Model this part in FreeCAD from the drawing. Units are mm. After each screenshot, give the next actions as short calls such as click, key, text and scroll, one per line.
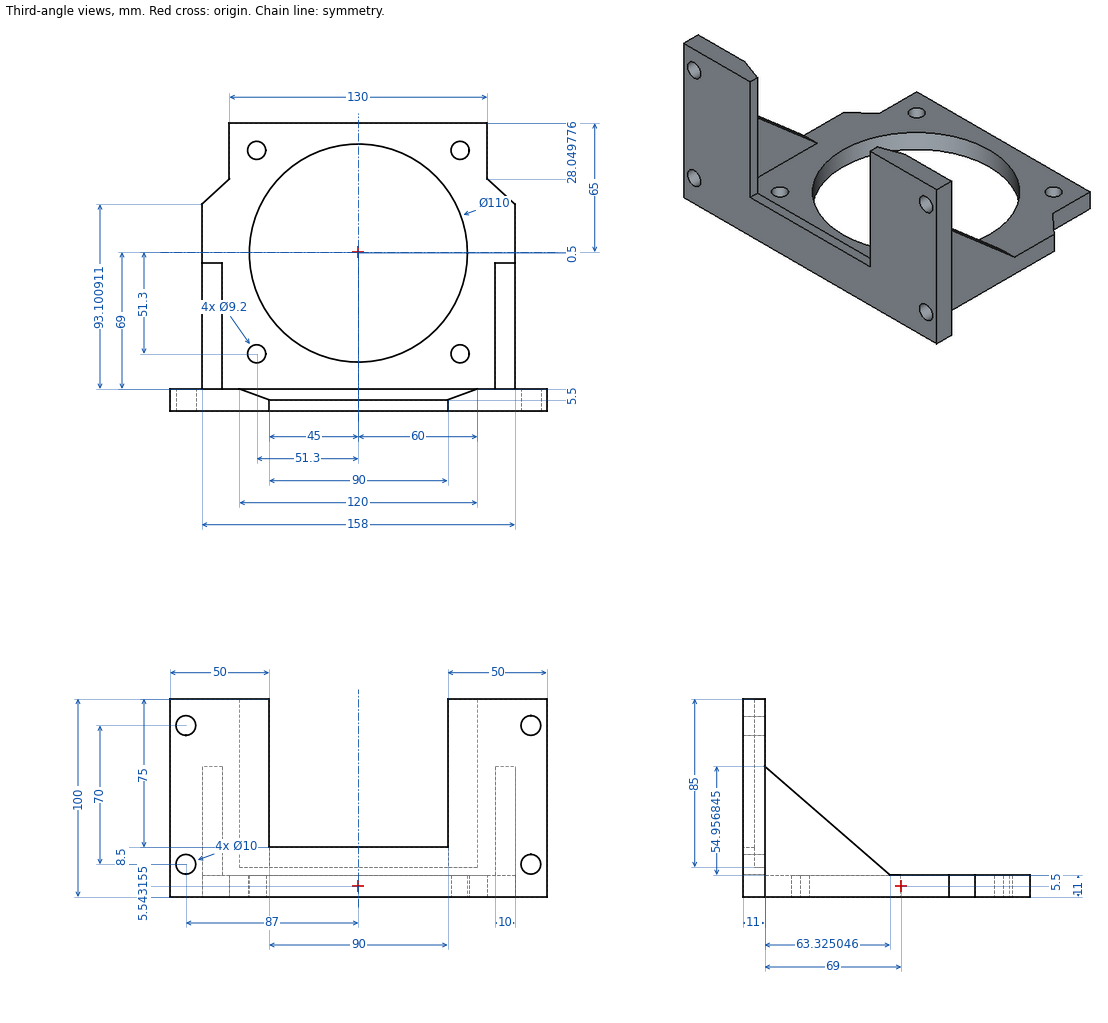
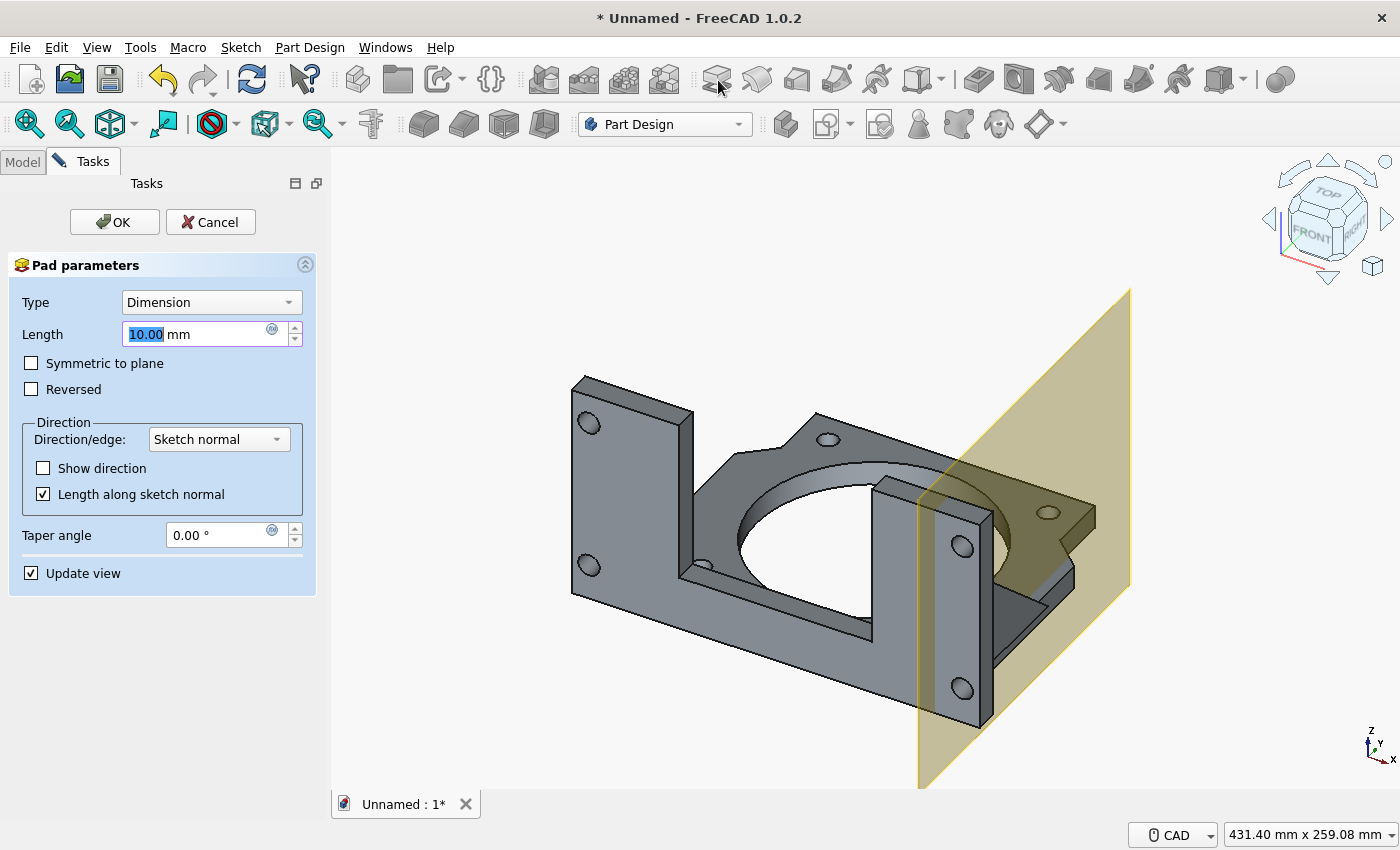
text(10)
key(Tab)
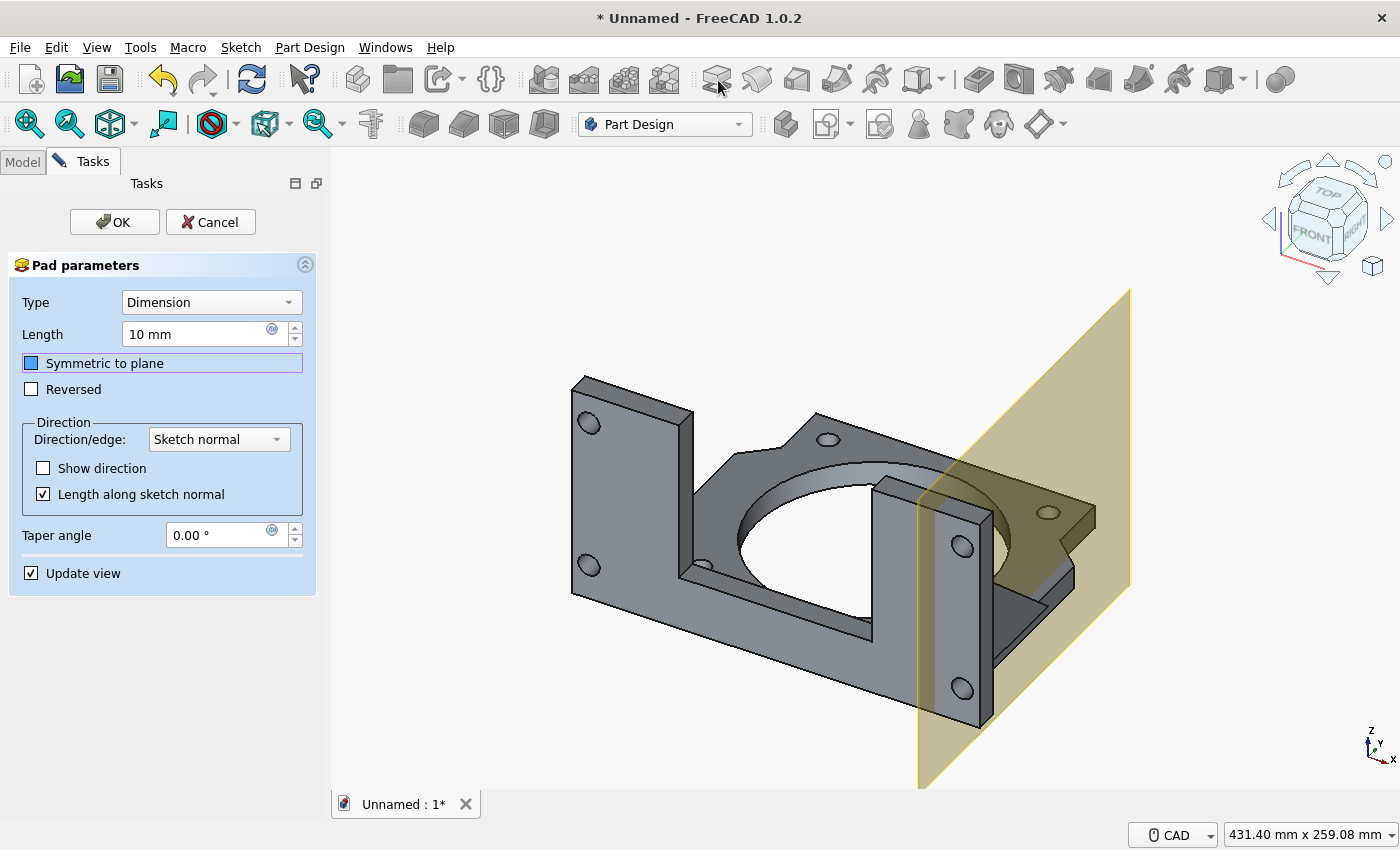
click(30, 363)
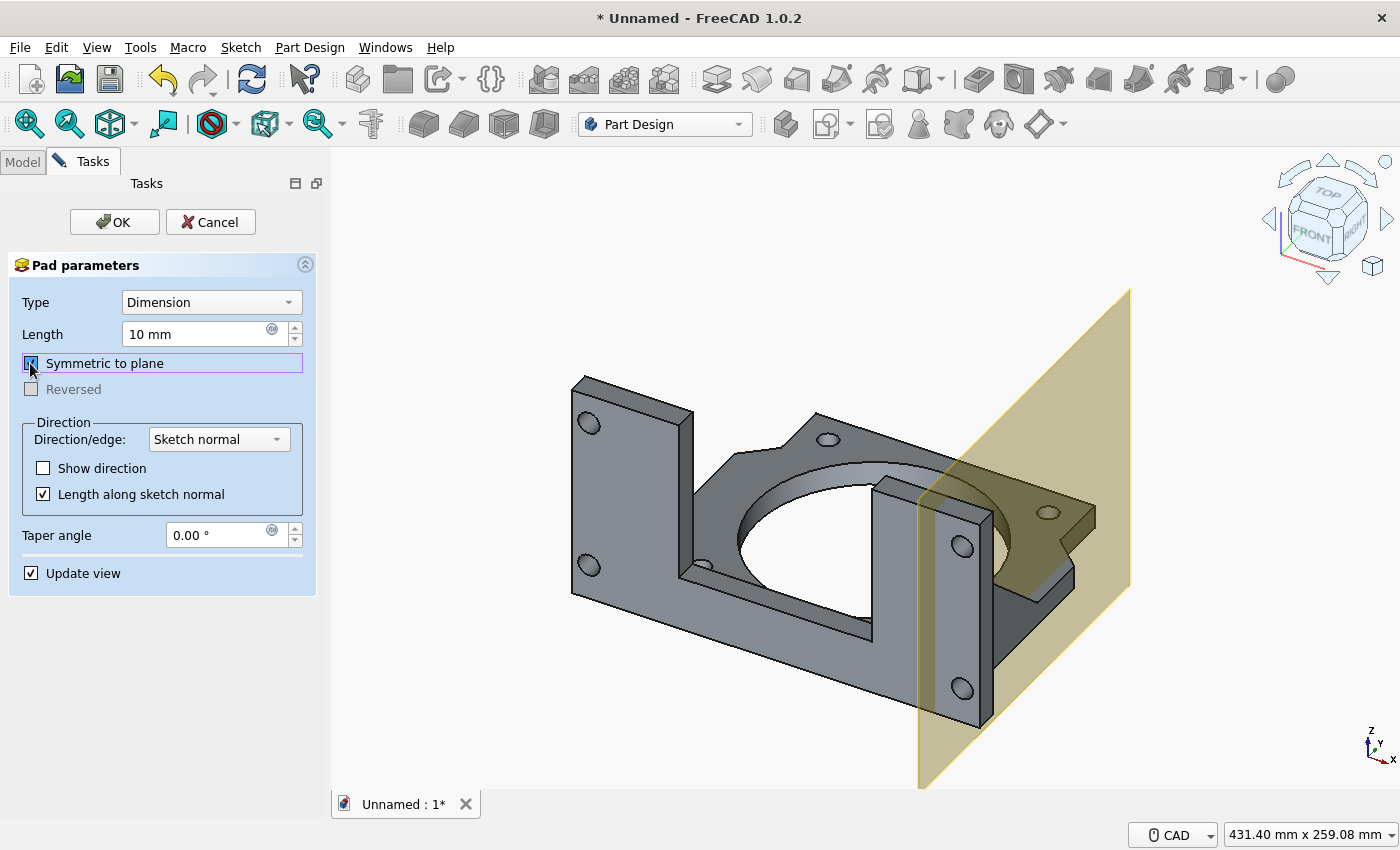
click(115, 222)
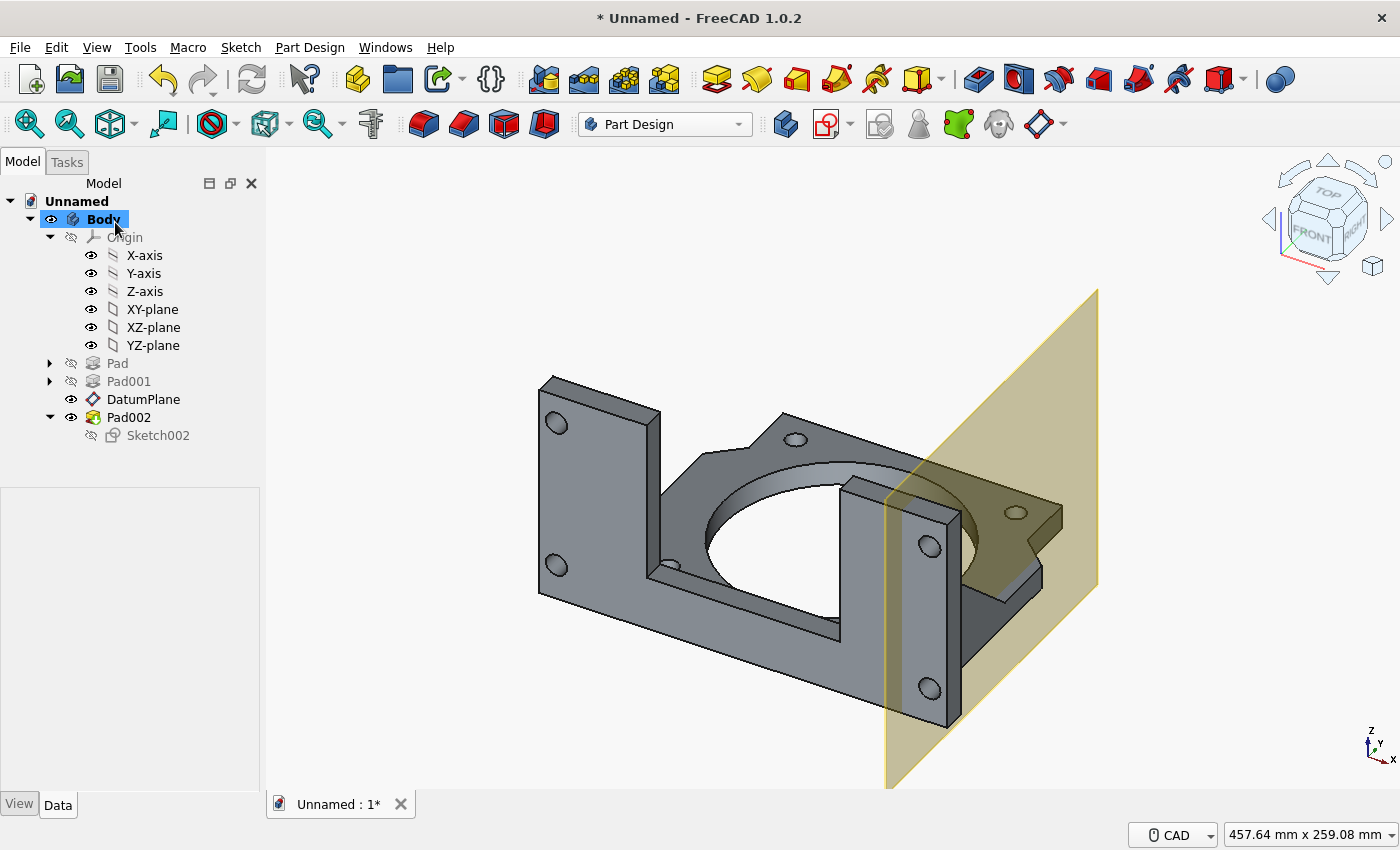
click(116, 399)
key(space)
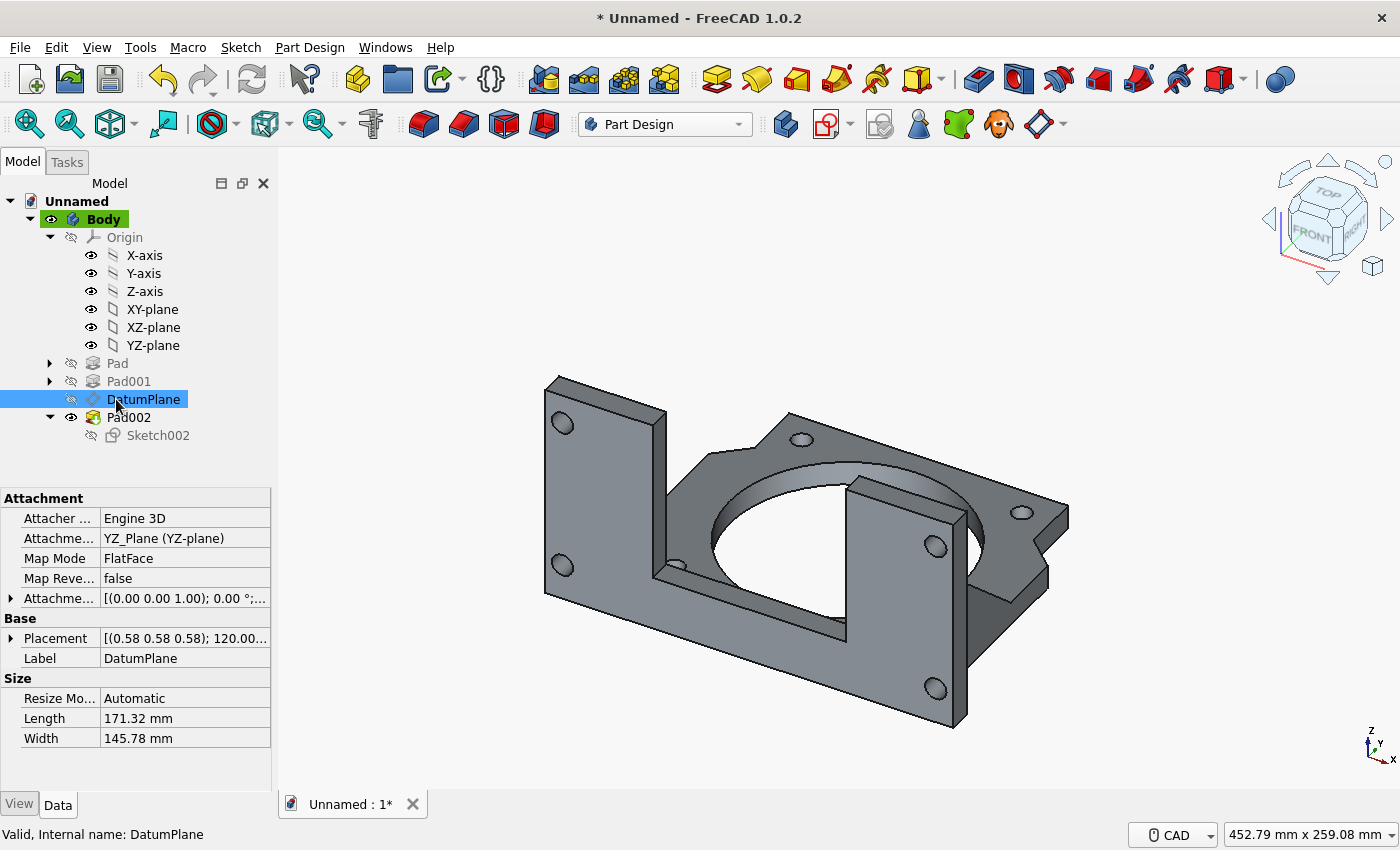
click(116, 417)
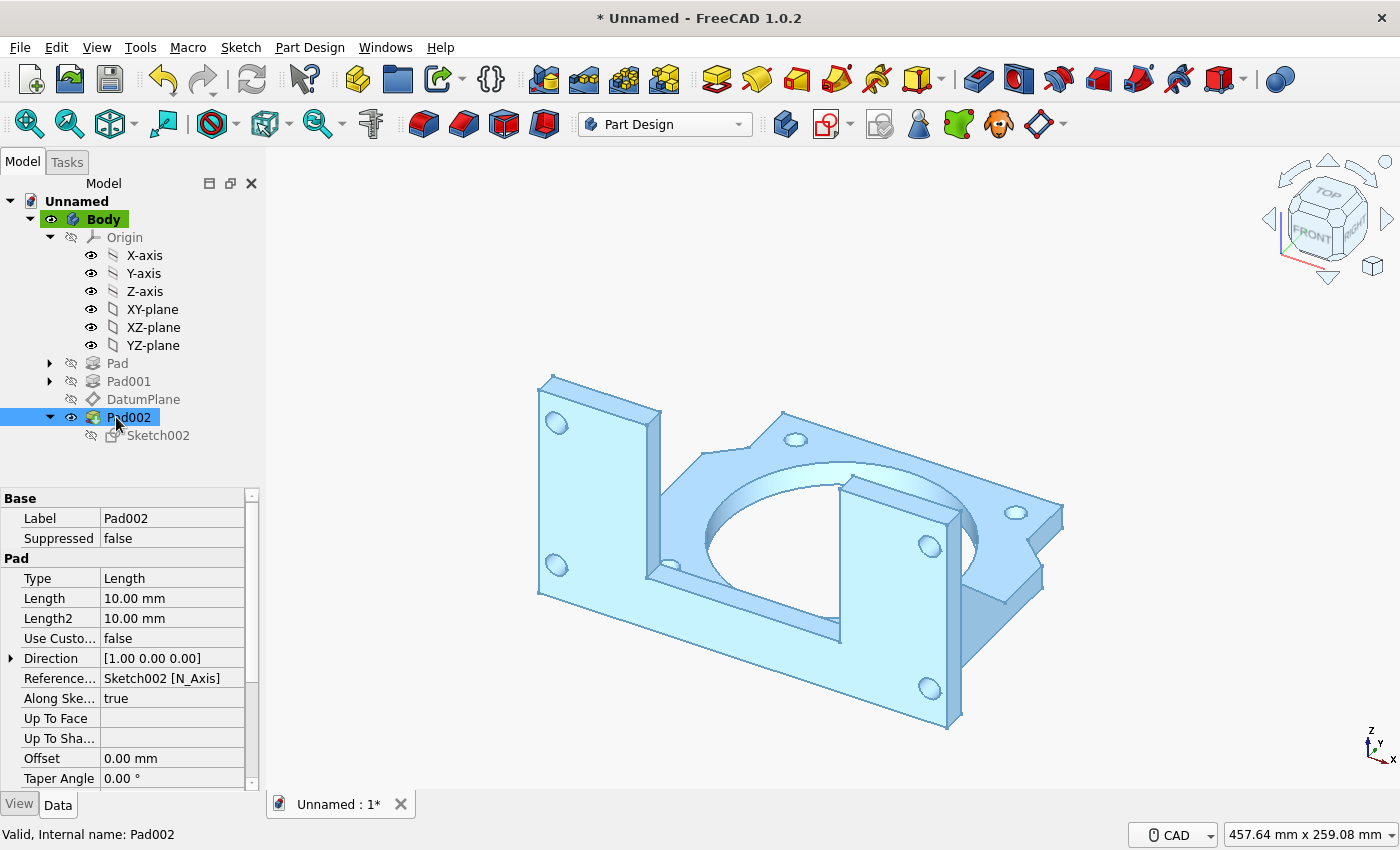
click(544, 80)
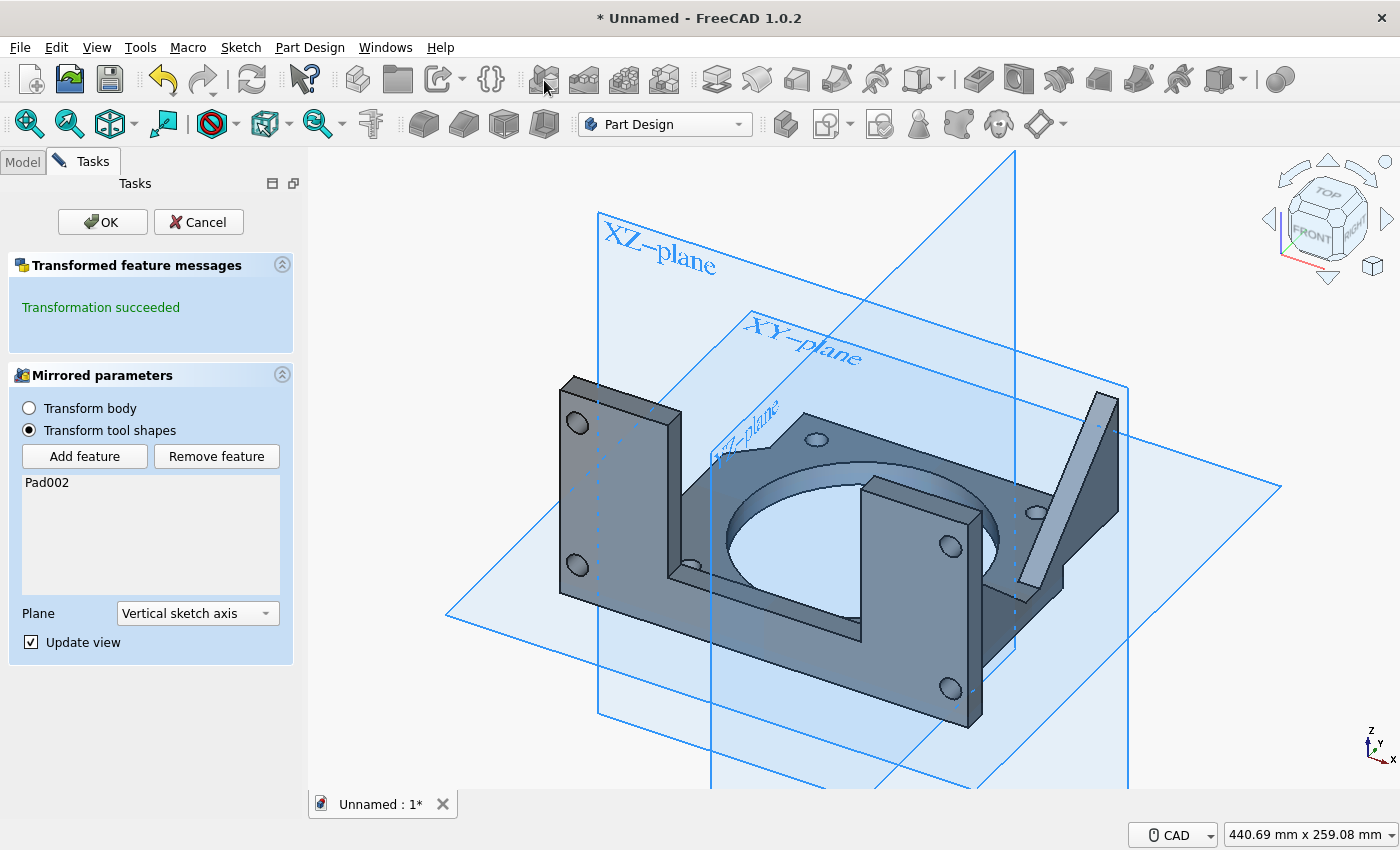
click(198, 614)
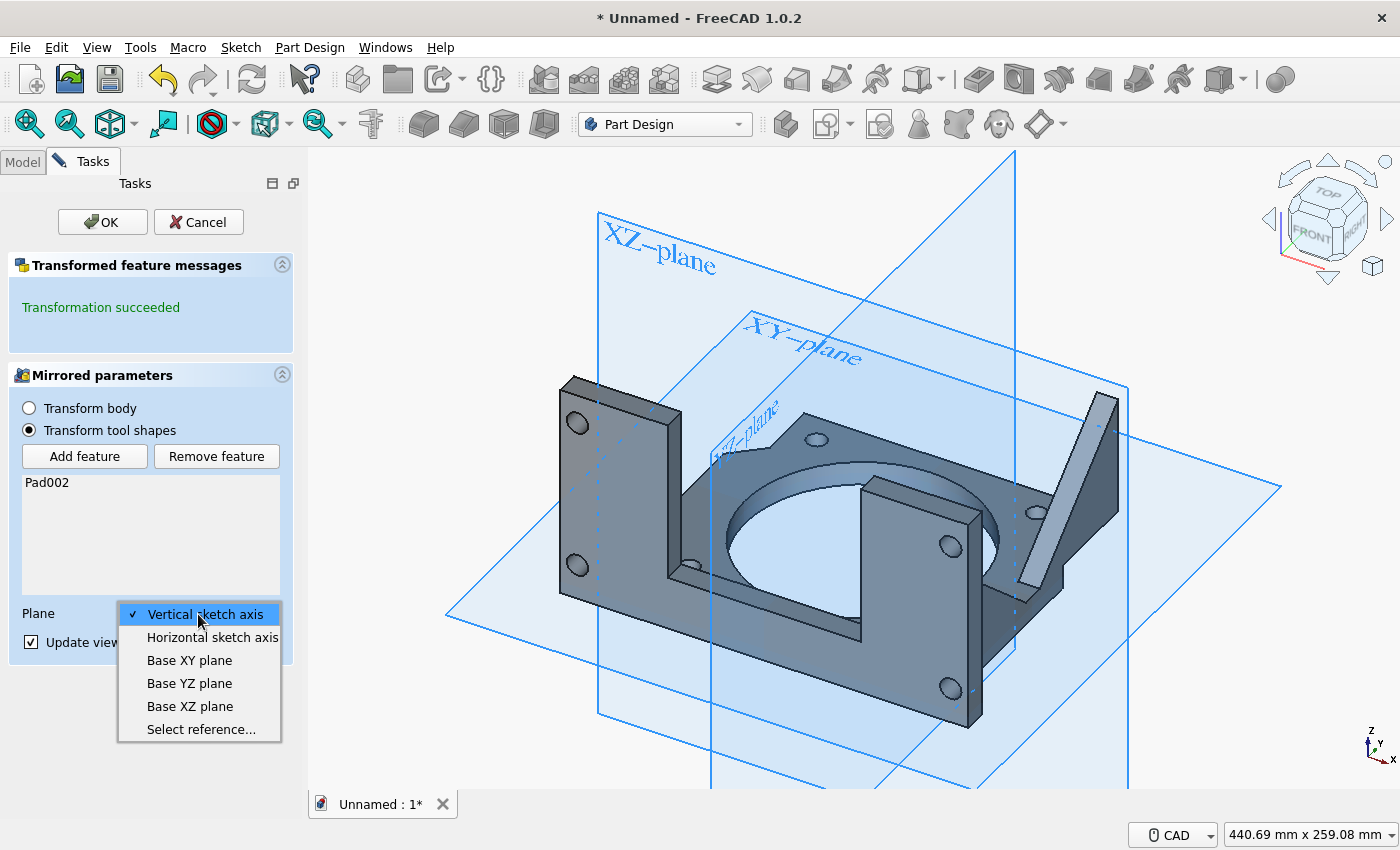
click(198, 684)